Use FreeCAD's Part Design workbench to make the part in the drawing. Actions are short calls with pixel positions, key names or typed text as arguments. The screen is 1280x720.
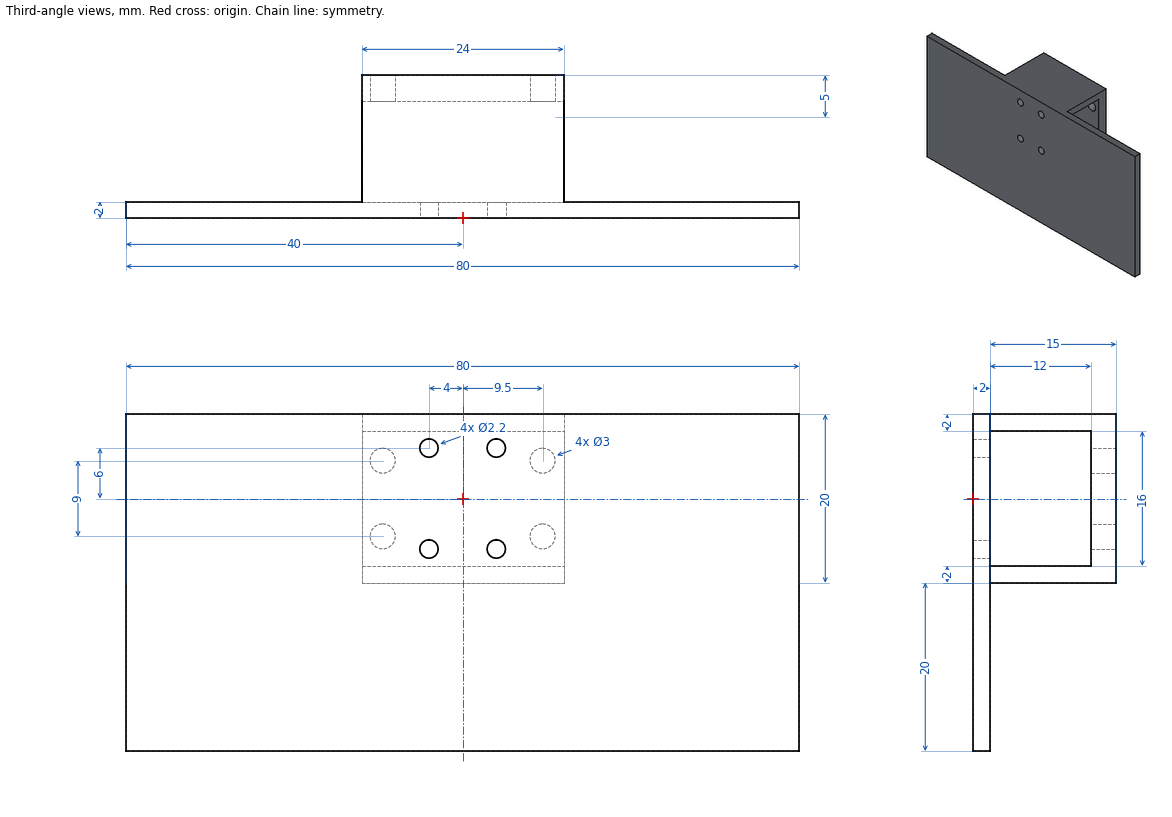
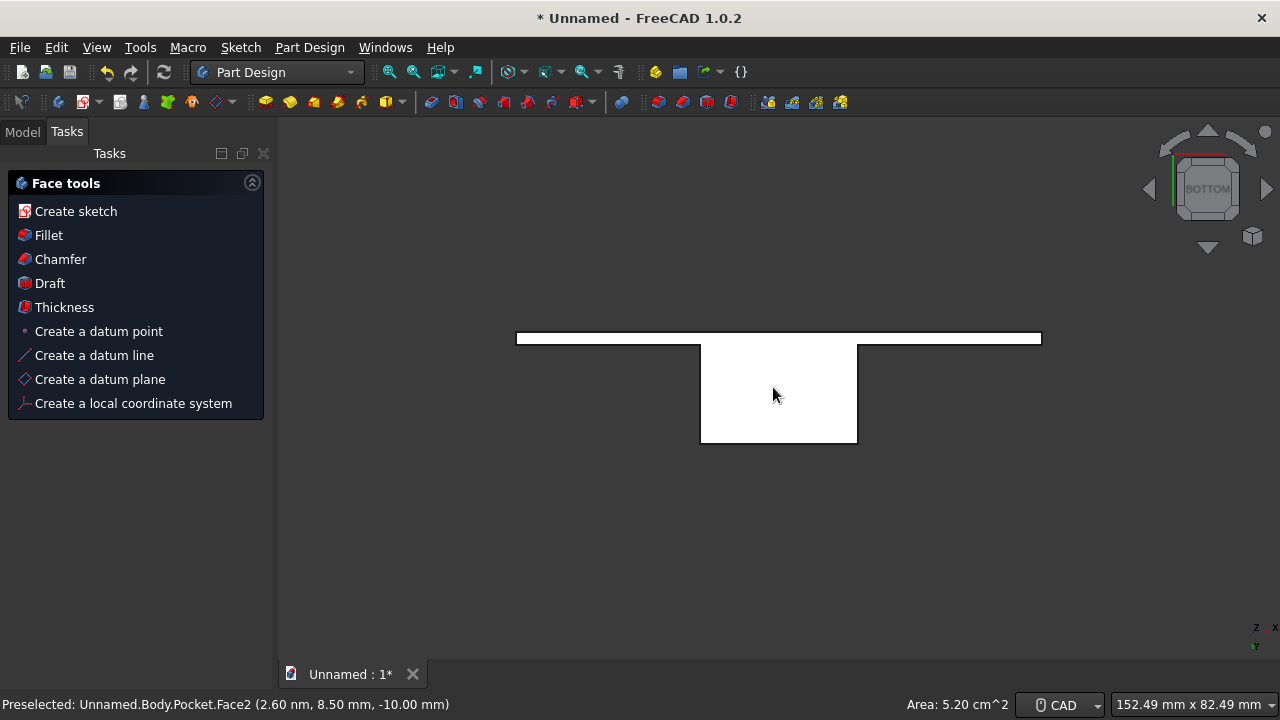
click(84, 102)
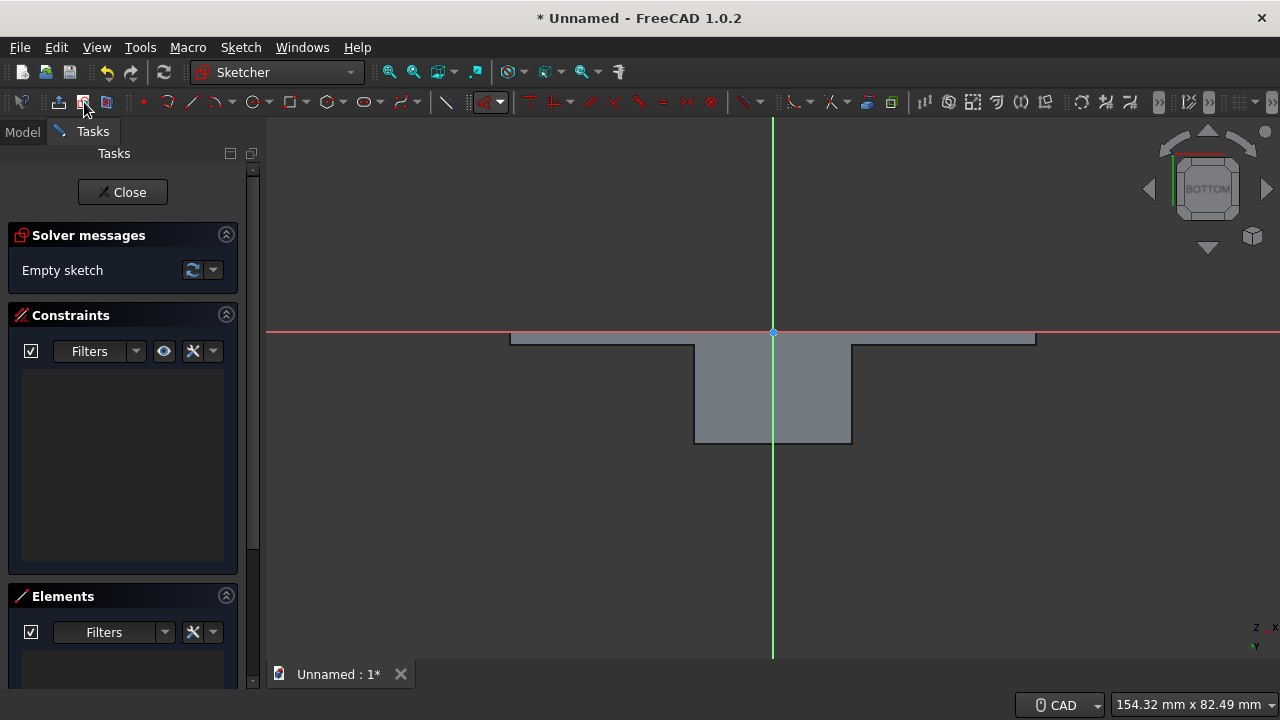
click(290, 102)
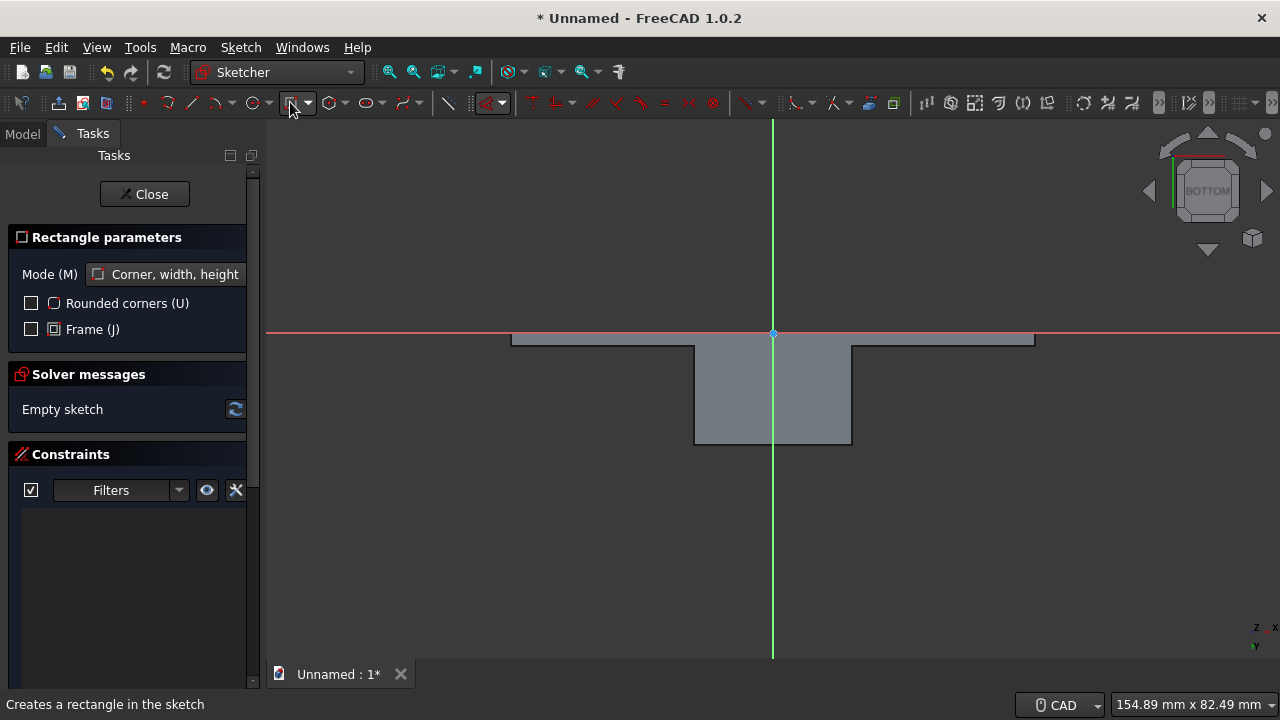
click(511, 333)
click(1035, 346)
key(Escape)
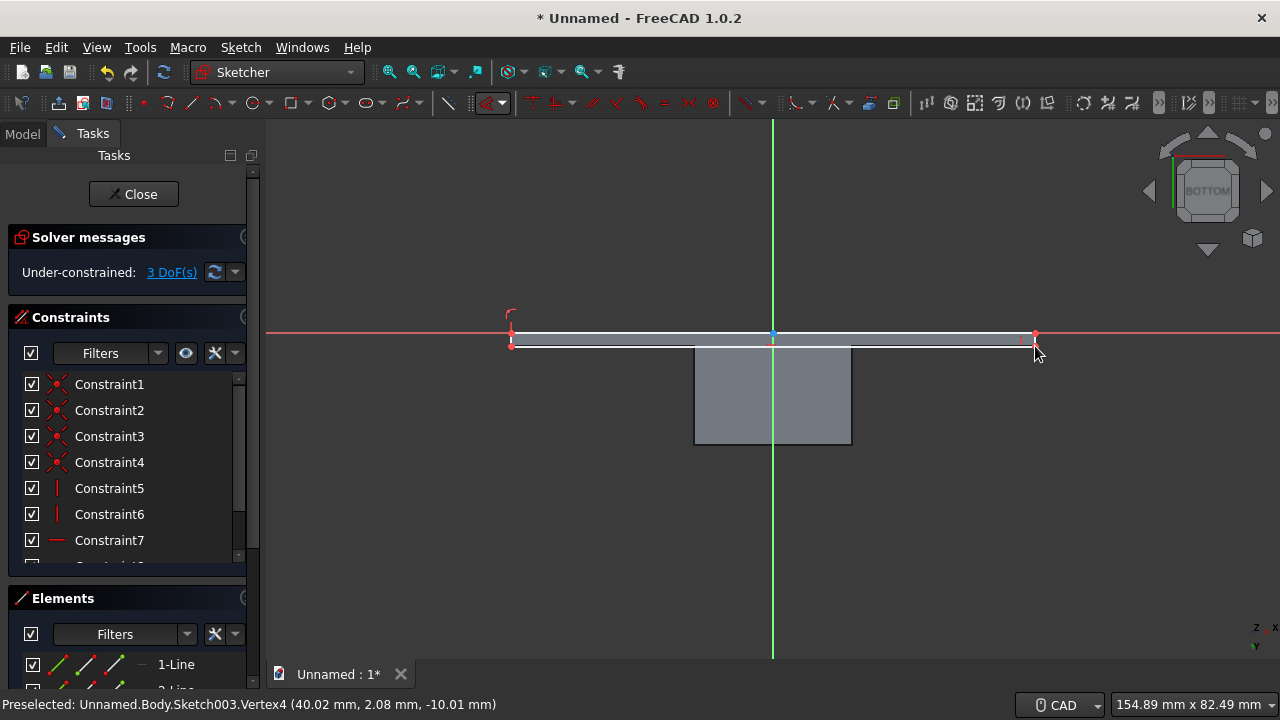
scroll(511, 340, up, 6)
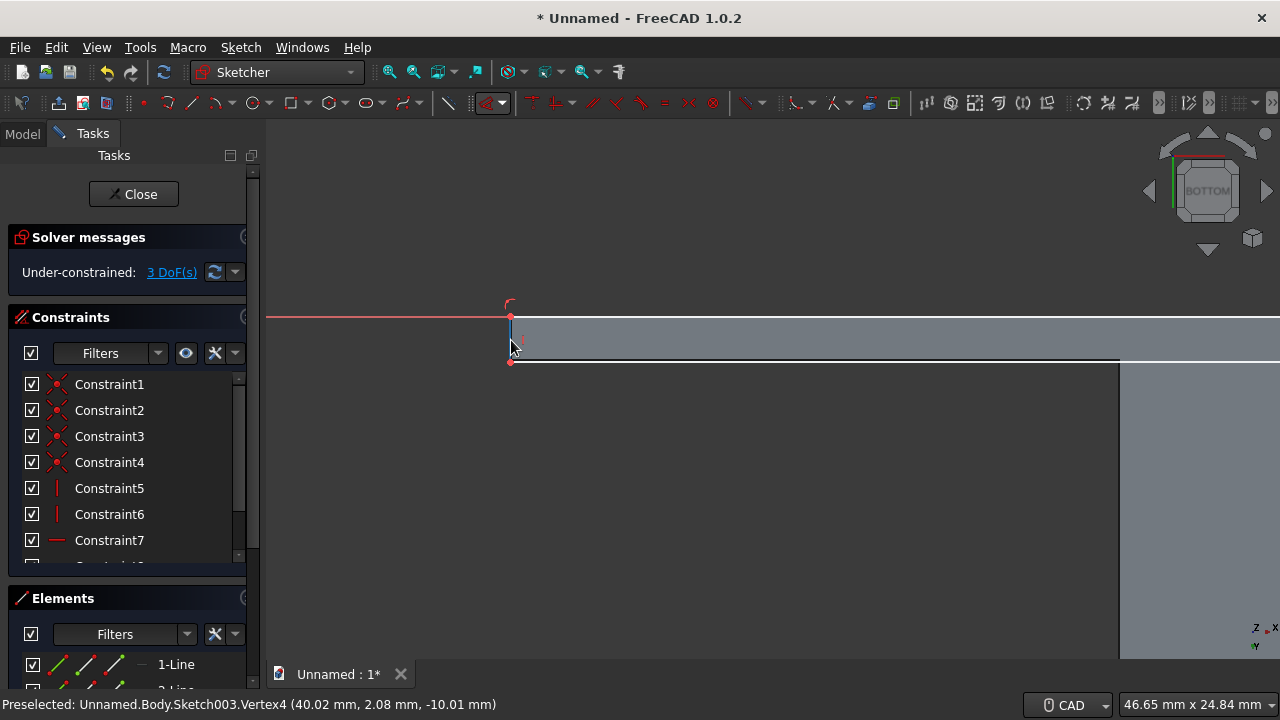
click(510, 340)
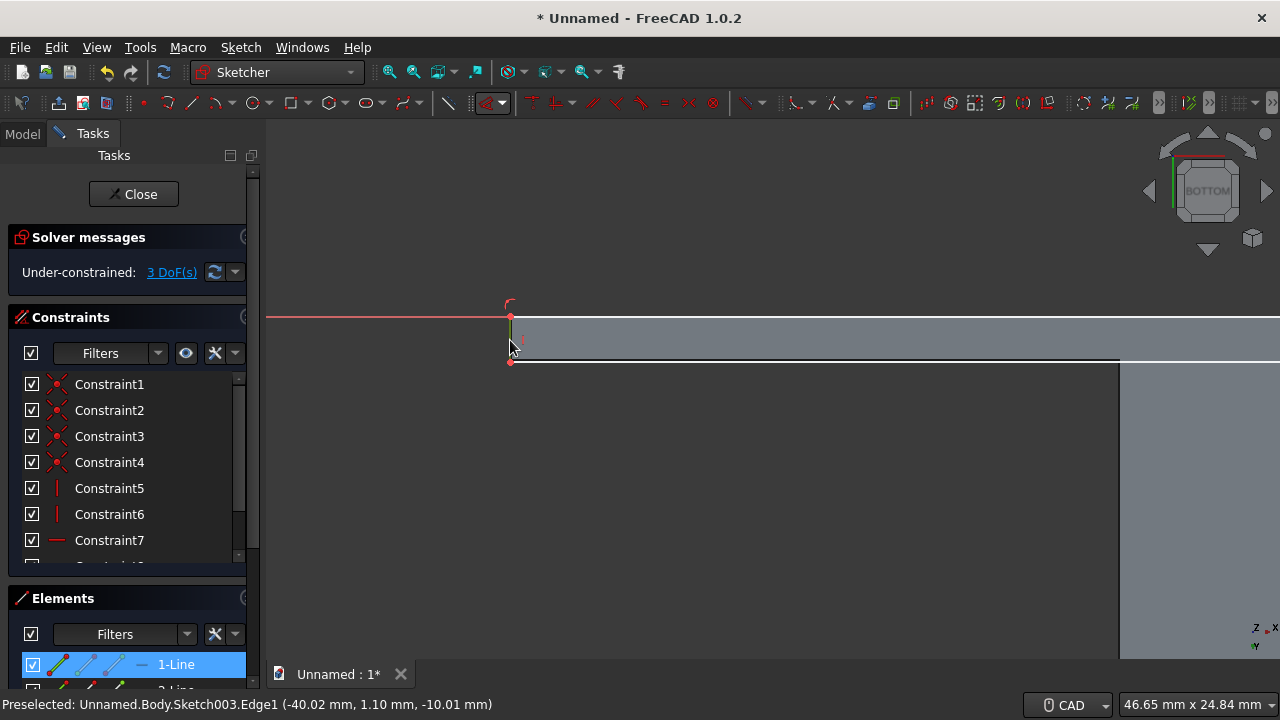
click(504, 104)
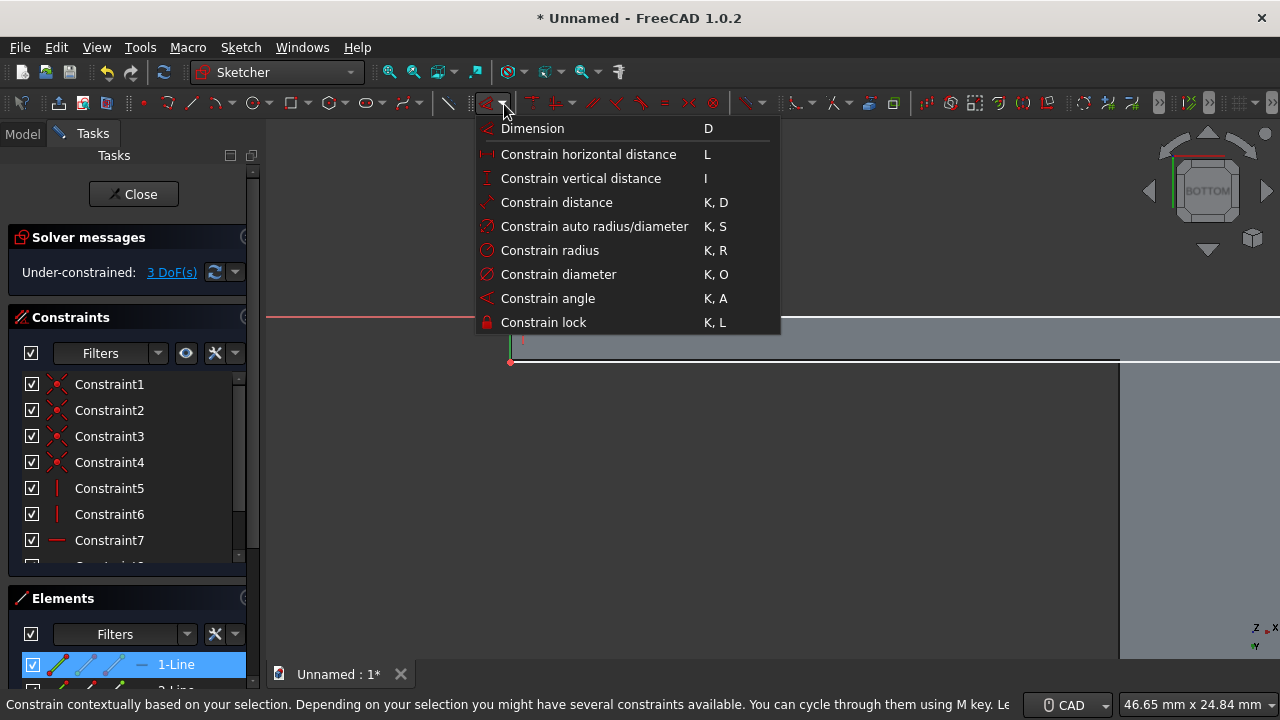
click(628, 178)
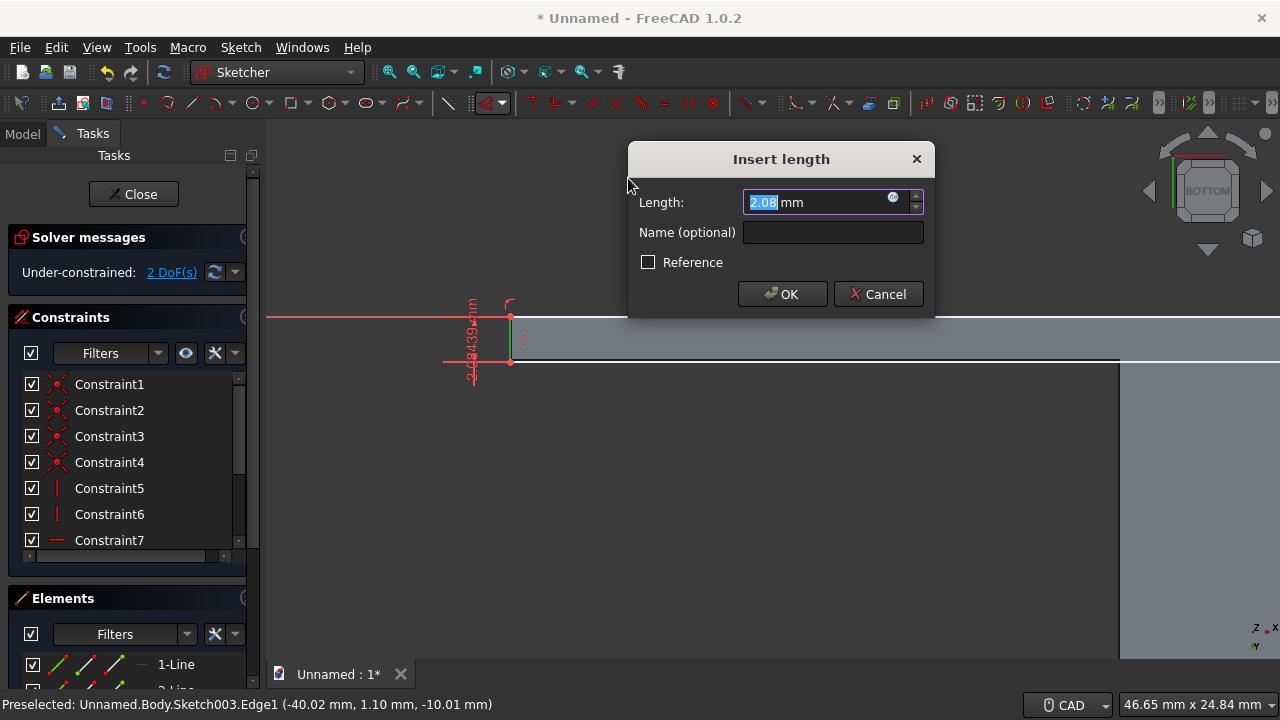
text(2)
key(Return)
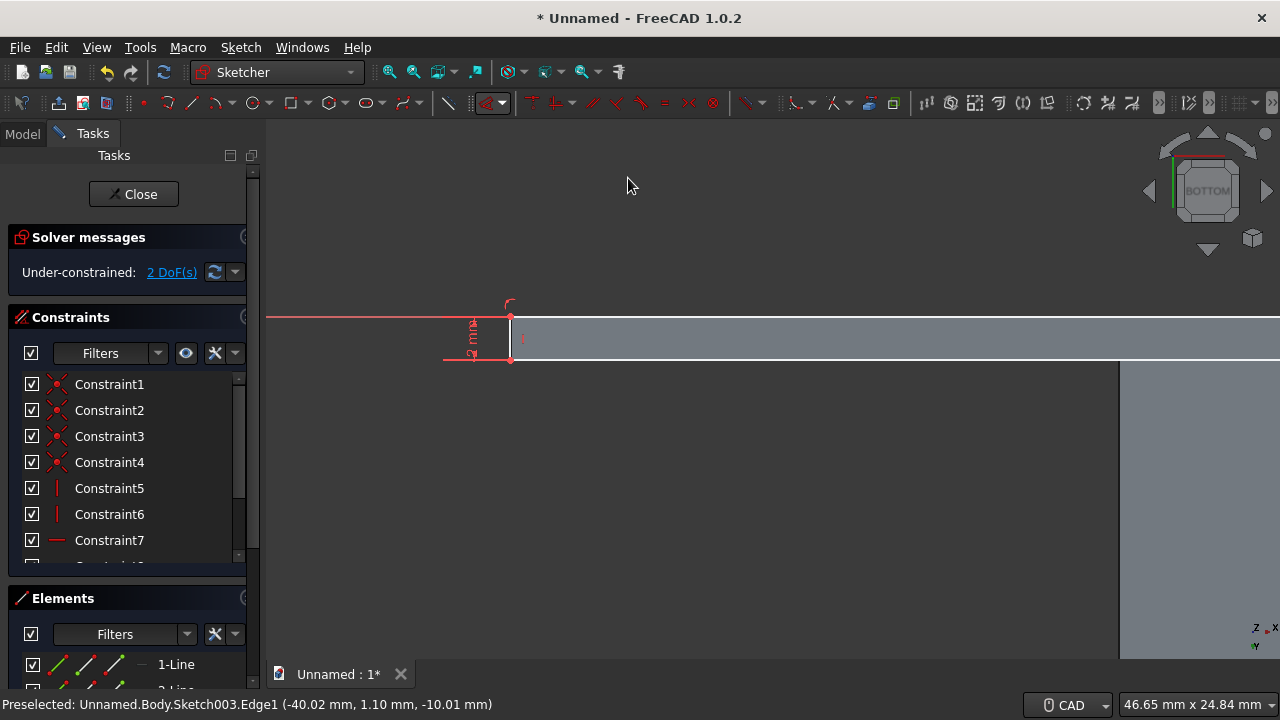
click(1032, 360)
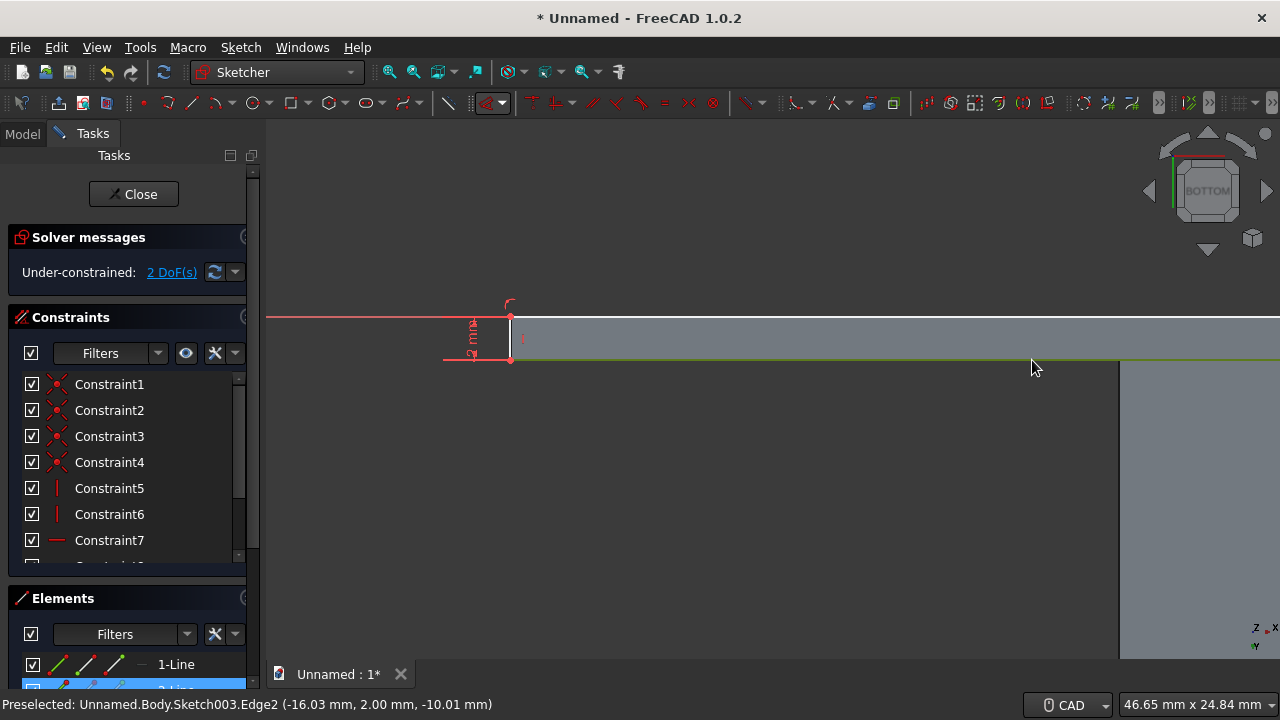
click(504, 104)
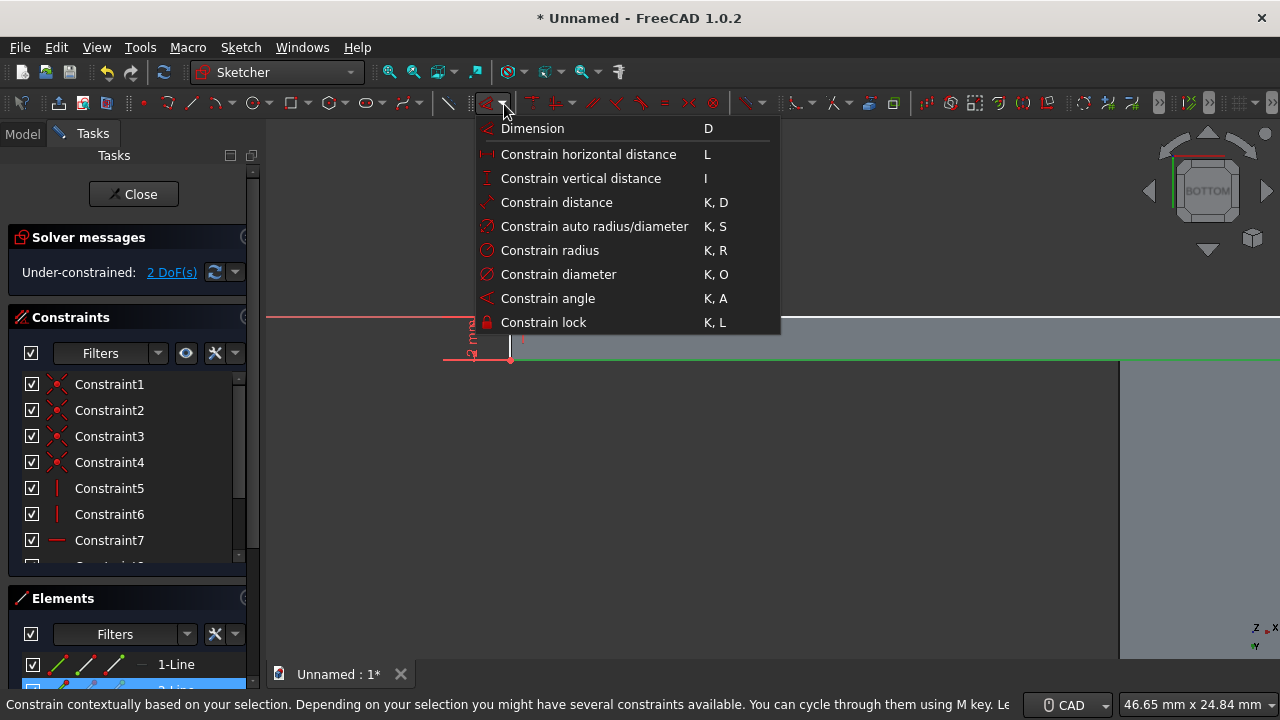
click(628, 154)